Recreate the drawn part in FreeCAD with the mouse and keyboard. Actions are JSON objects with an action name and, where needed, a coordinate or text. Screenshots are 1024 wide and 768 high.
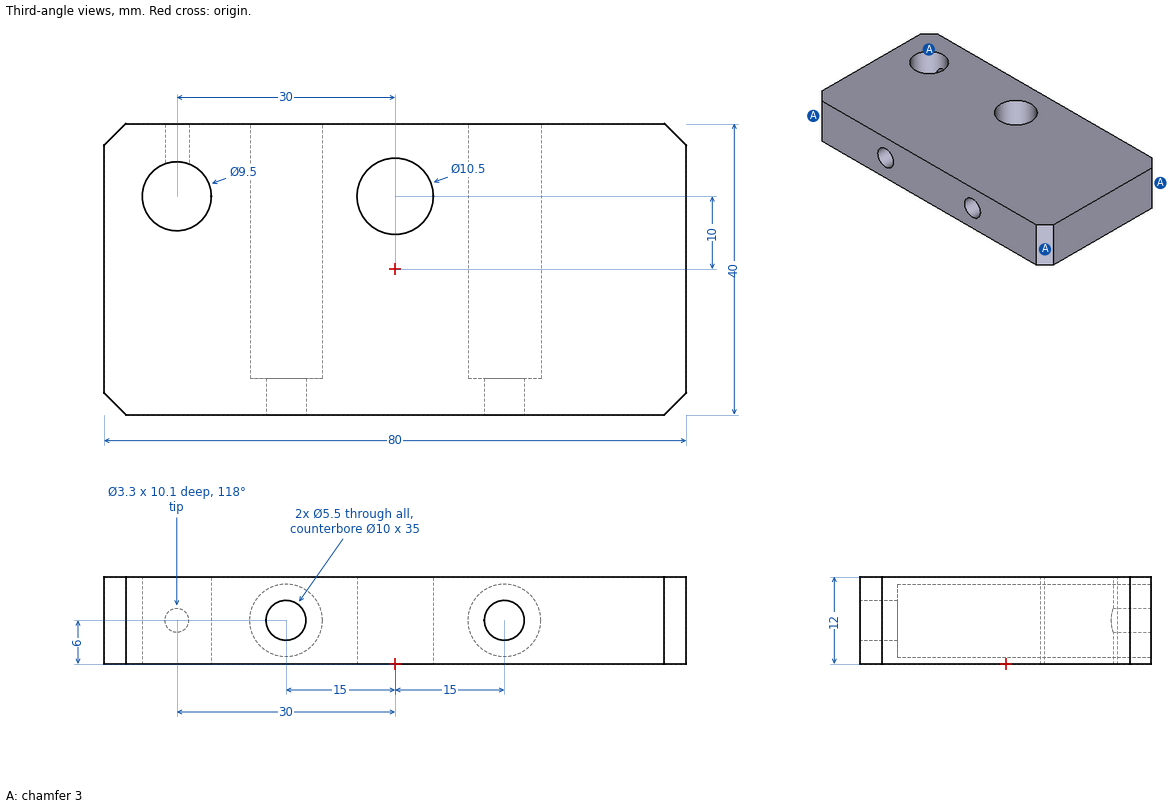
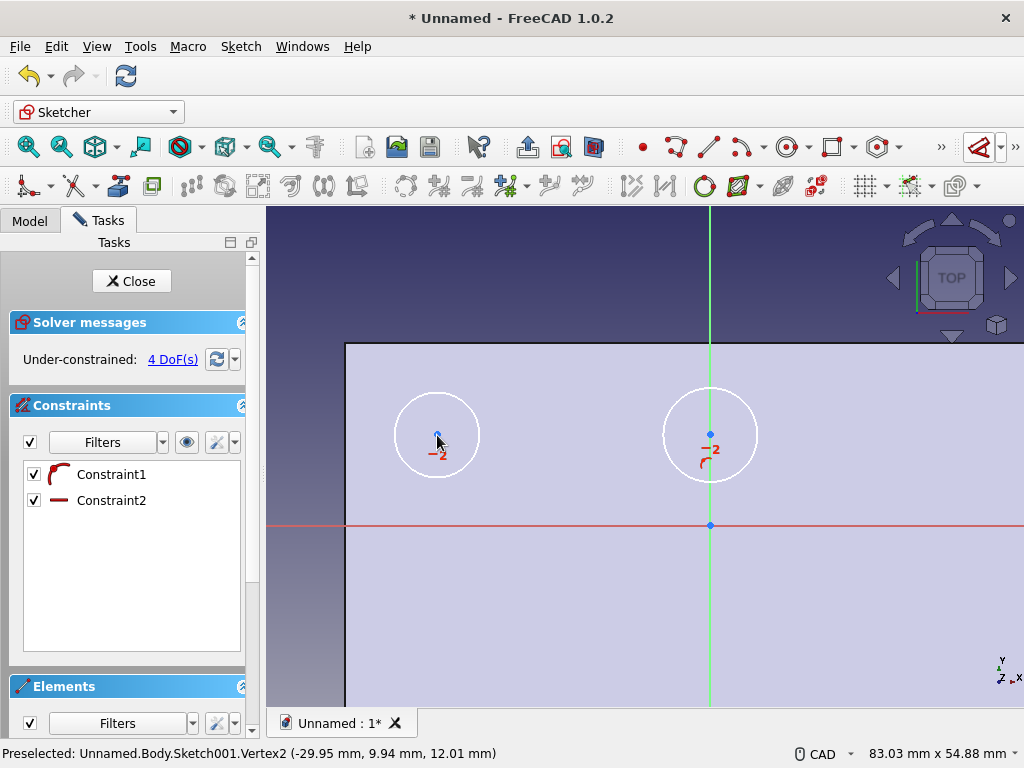
{"action": "left_click", "coordinate": [744, 402]}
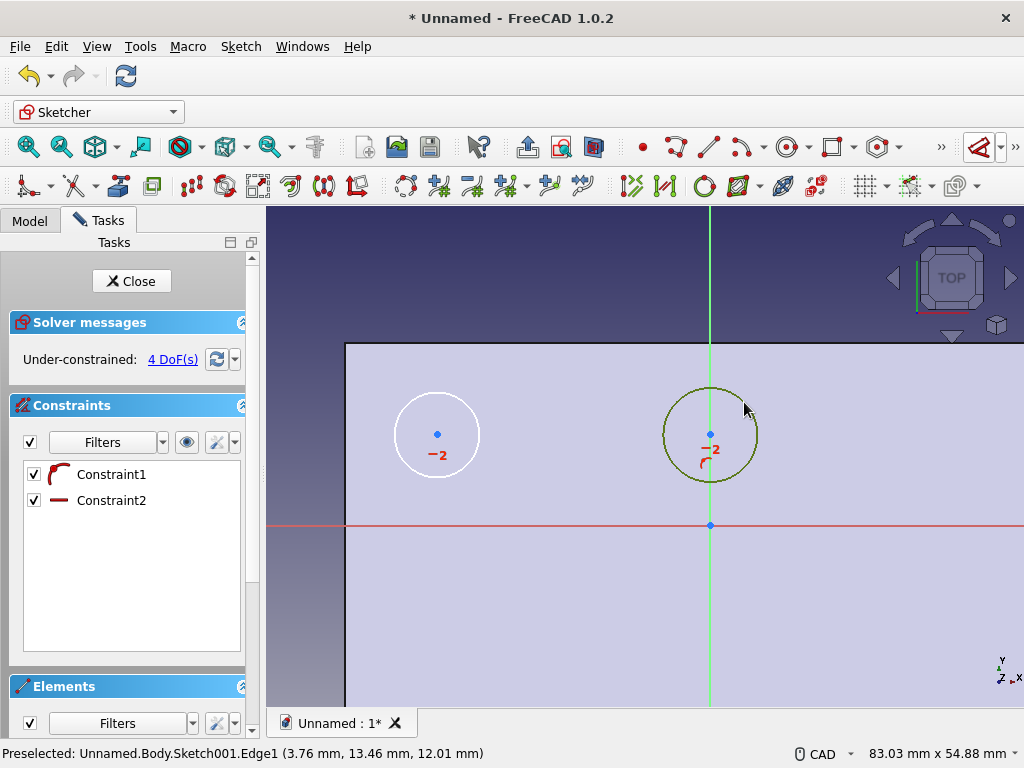
{"action": "key", "text": "k o"}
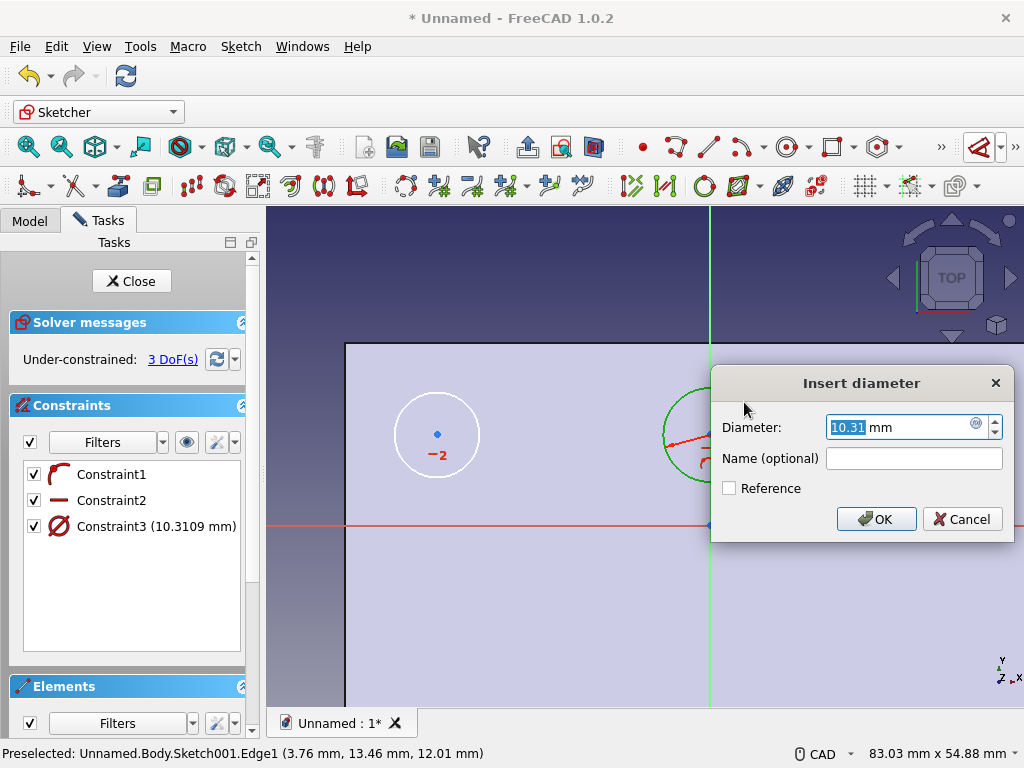
{"action": "type", "text": "10.5"}
{"action": "key", "text": "Return"}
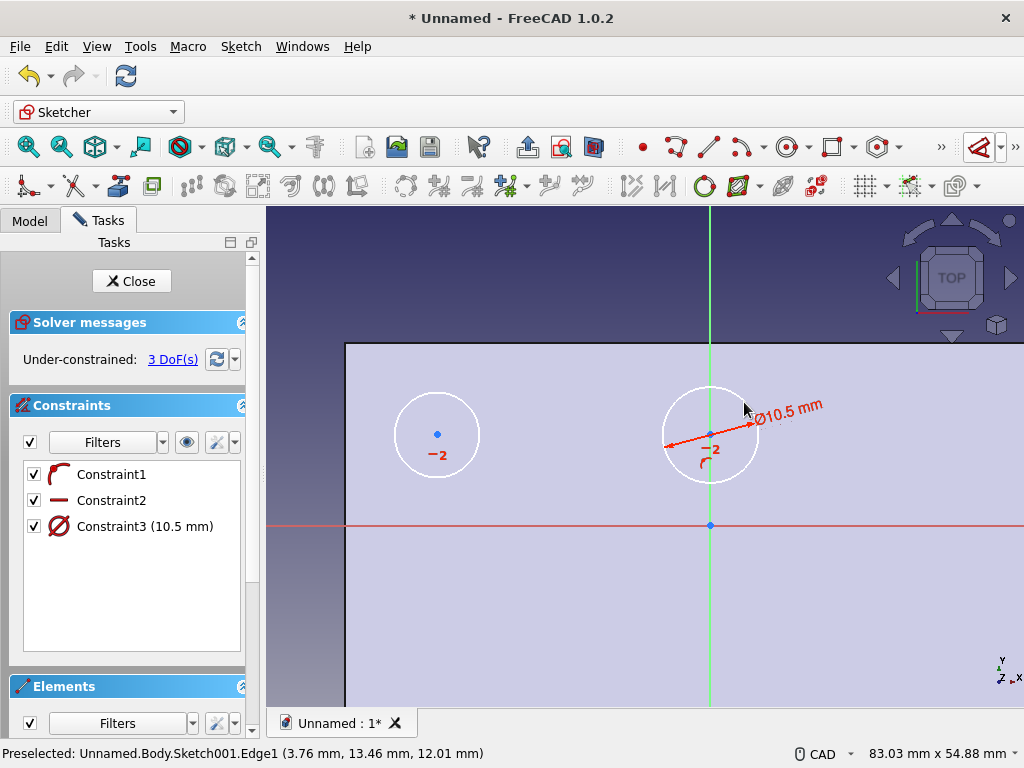
{"action": "left_click", "coordinate": [467, 405]}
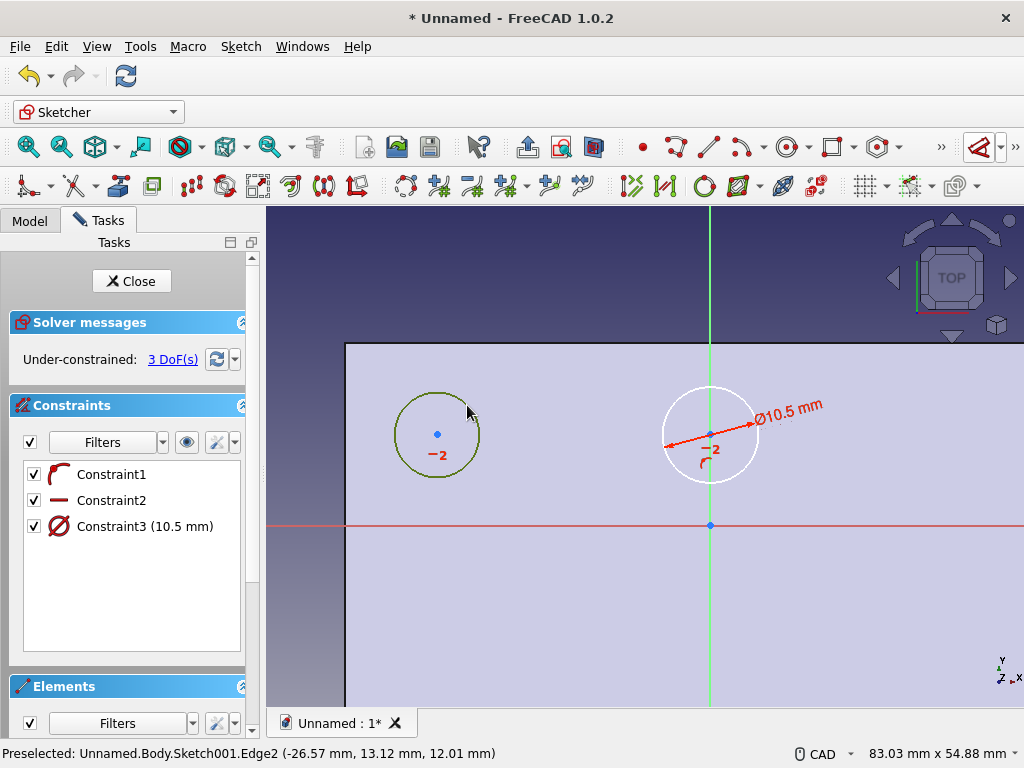
{"action": "key", "text": "k o"}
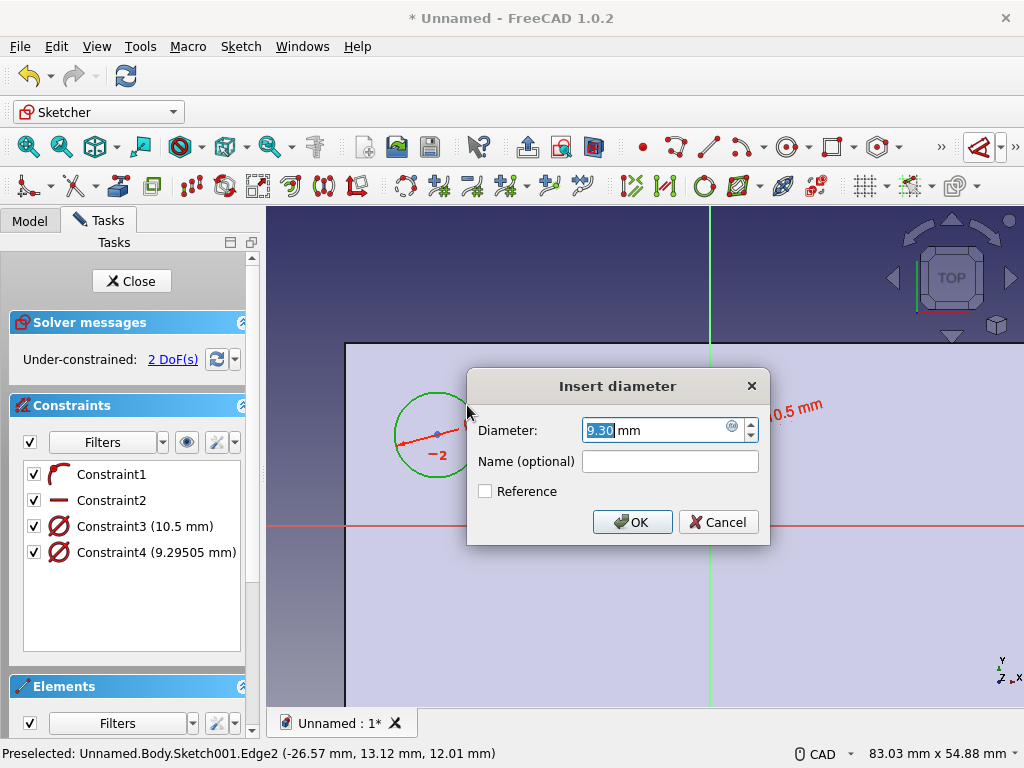
{"action": "type", "text": "9.5"}
{"action": "key", "text": "Return"}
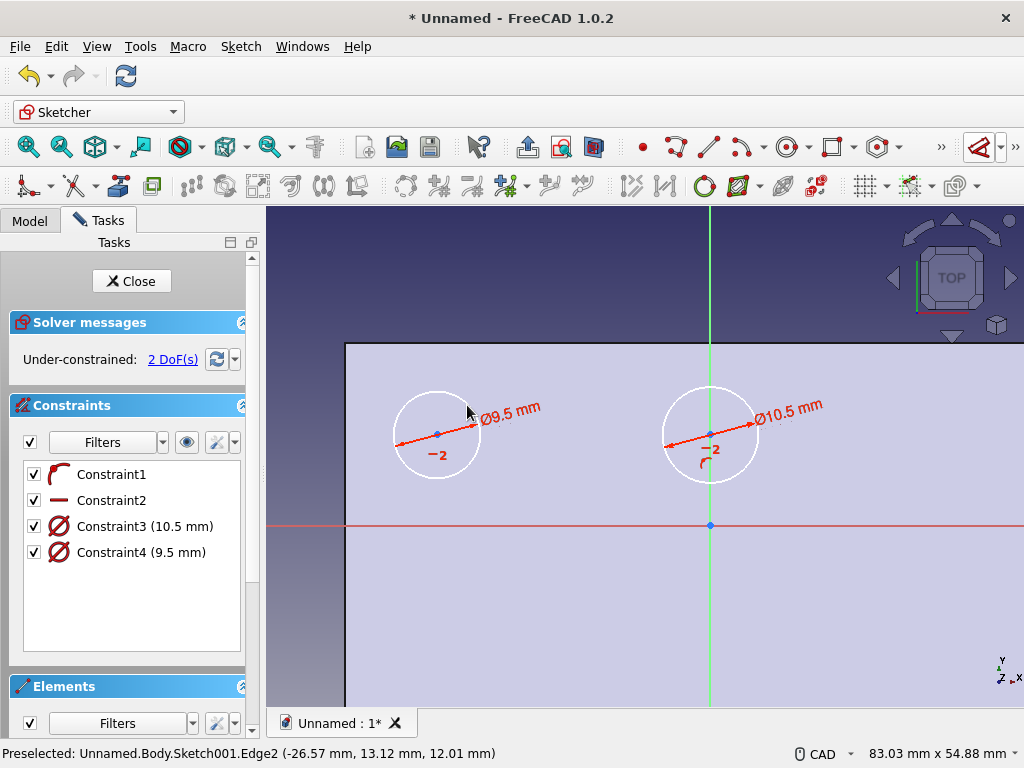
{"action": "left_click", "coordinate": [710, 435]}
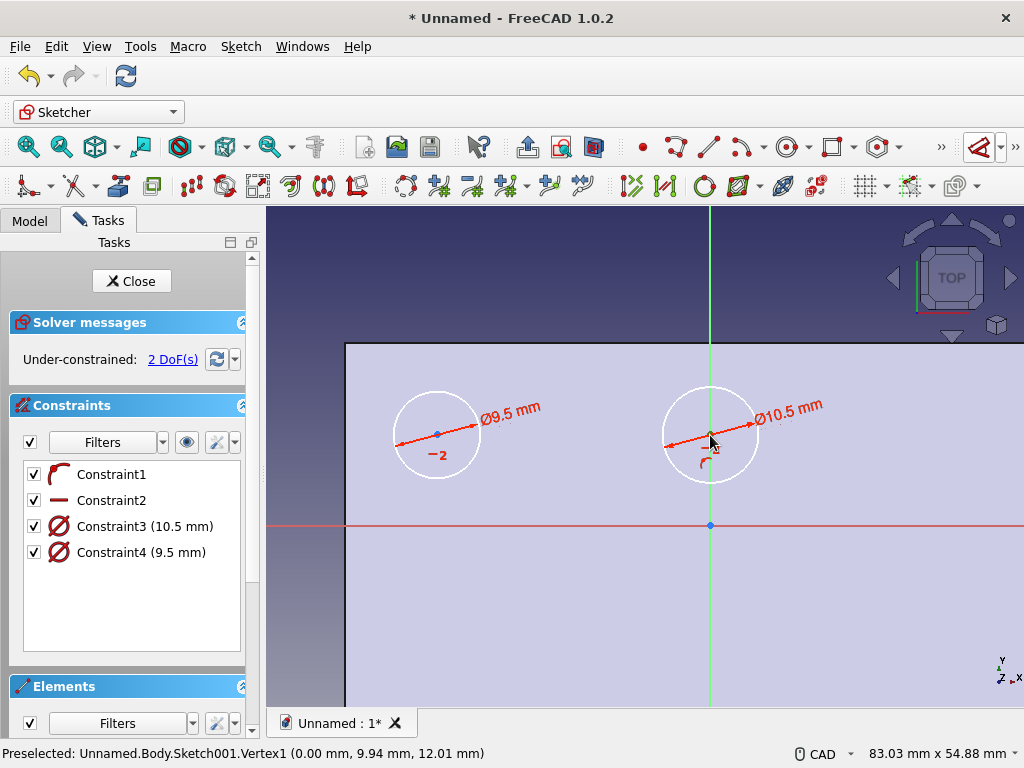
{"action": "key", "text": "i"}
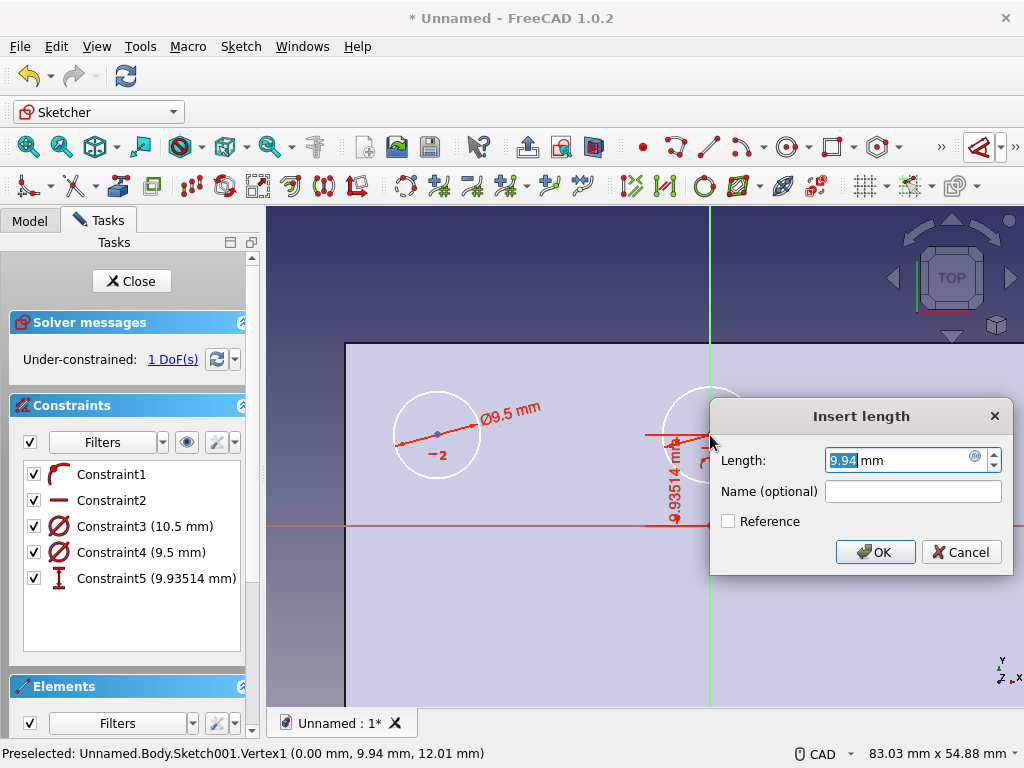
{"action": "type", "text": "10"}
{"action": "key", "text": "Return"}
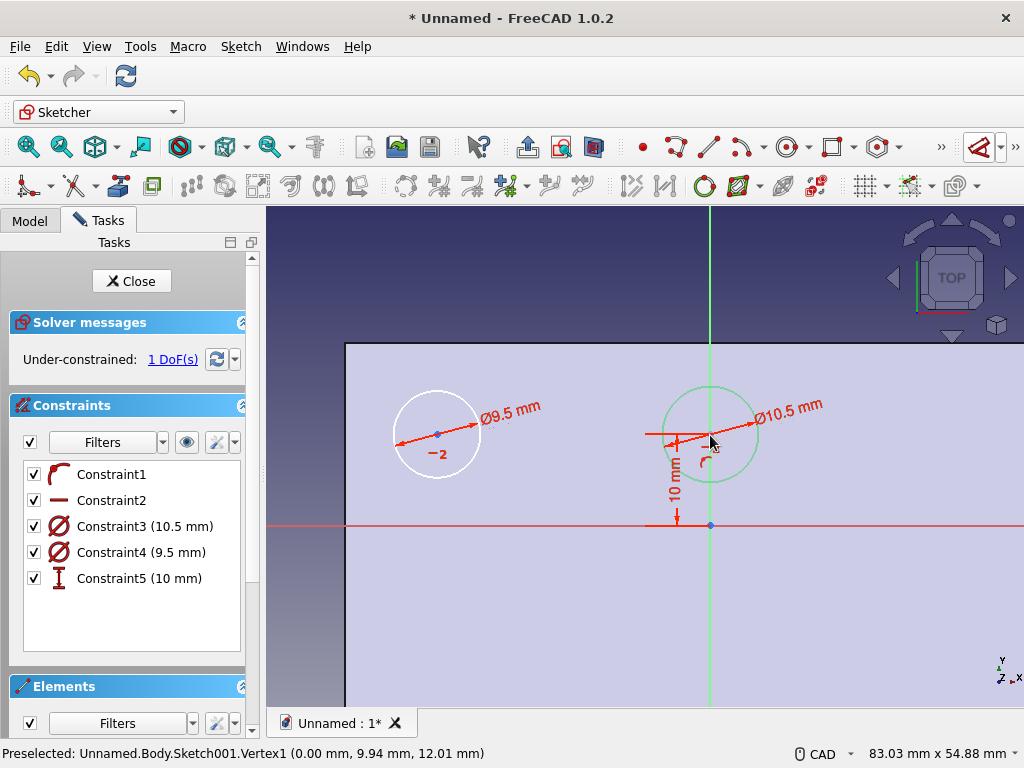
{"action": "left_click", "coordinate": [437, 434]}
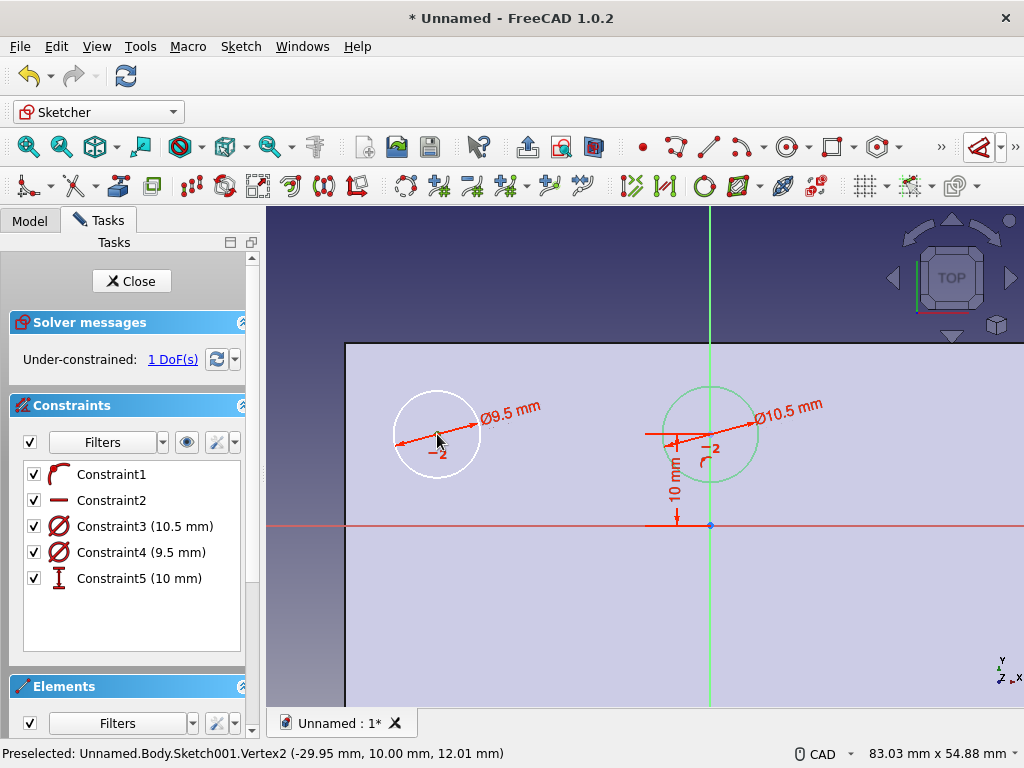
{"action": "key", "text": "l"}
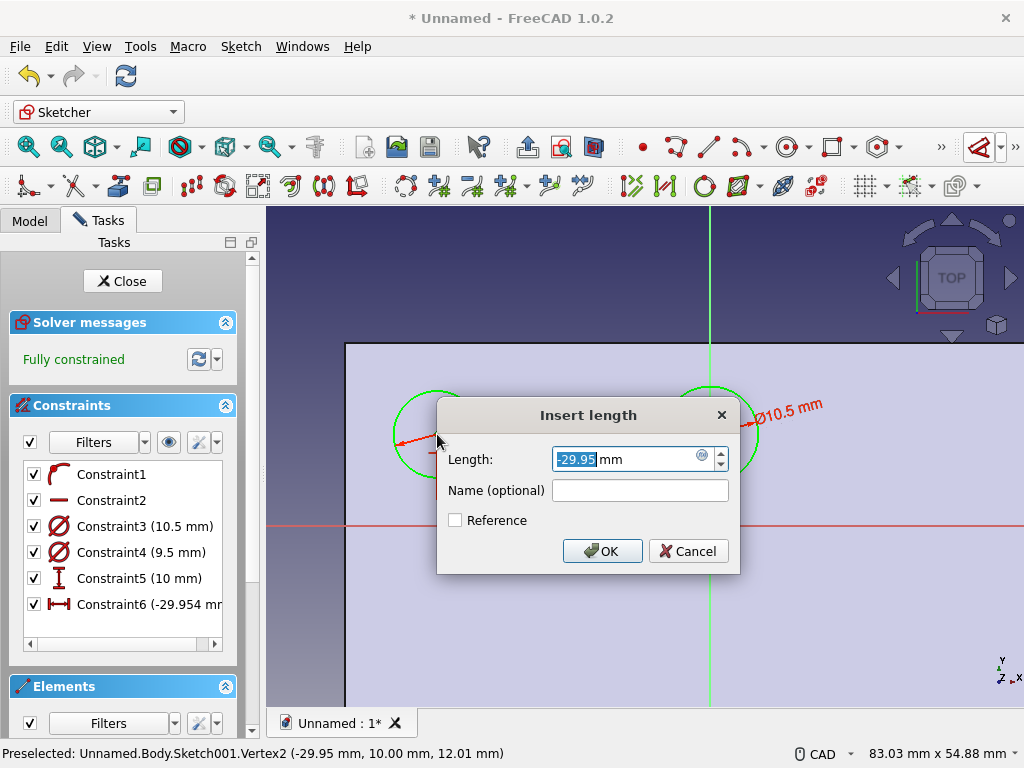
{"action": "type", "text": "-30"}
{"action": "key", "text": "Return"}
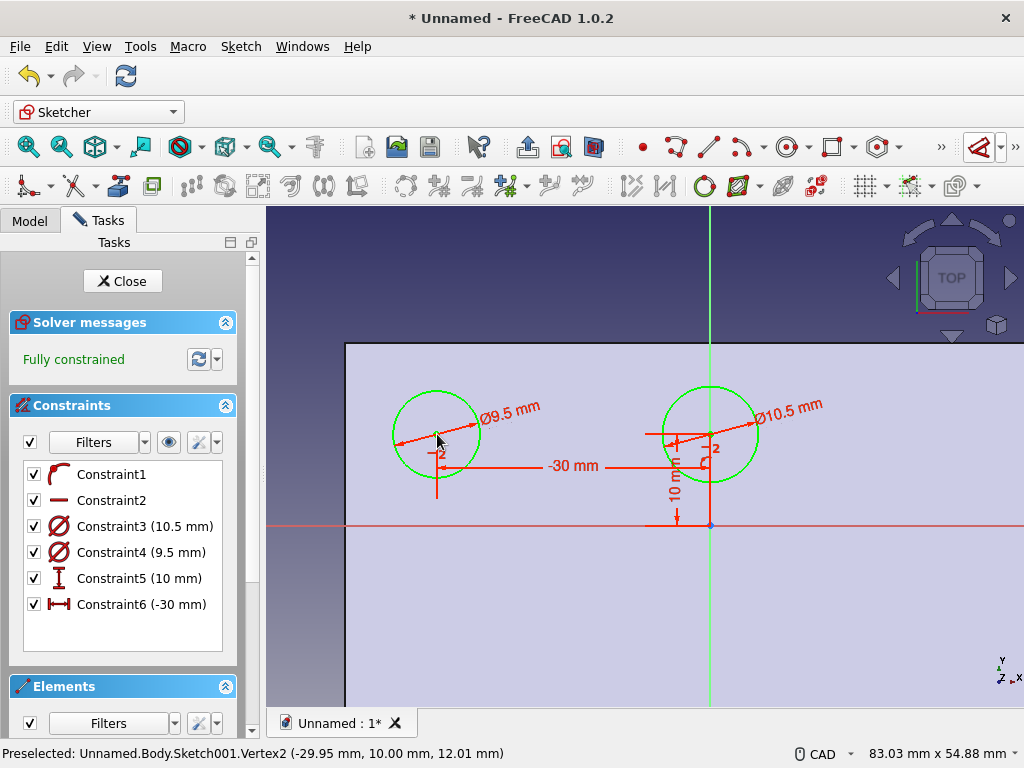
{"action": "left_click", "coordinate": [123, 281]}